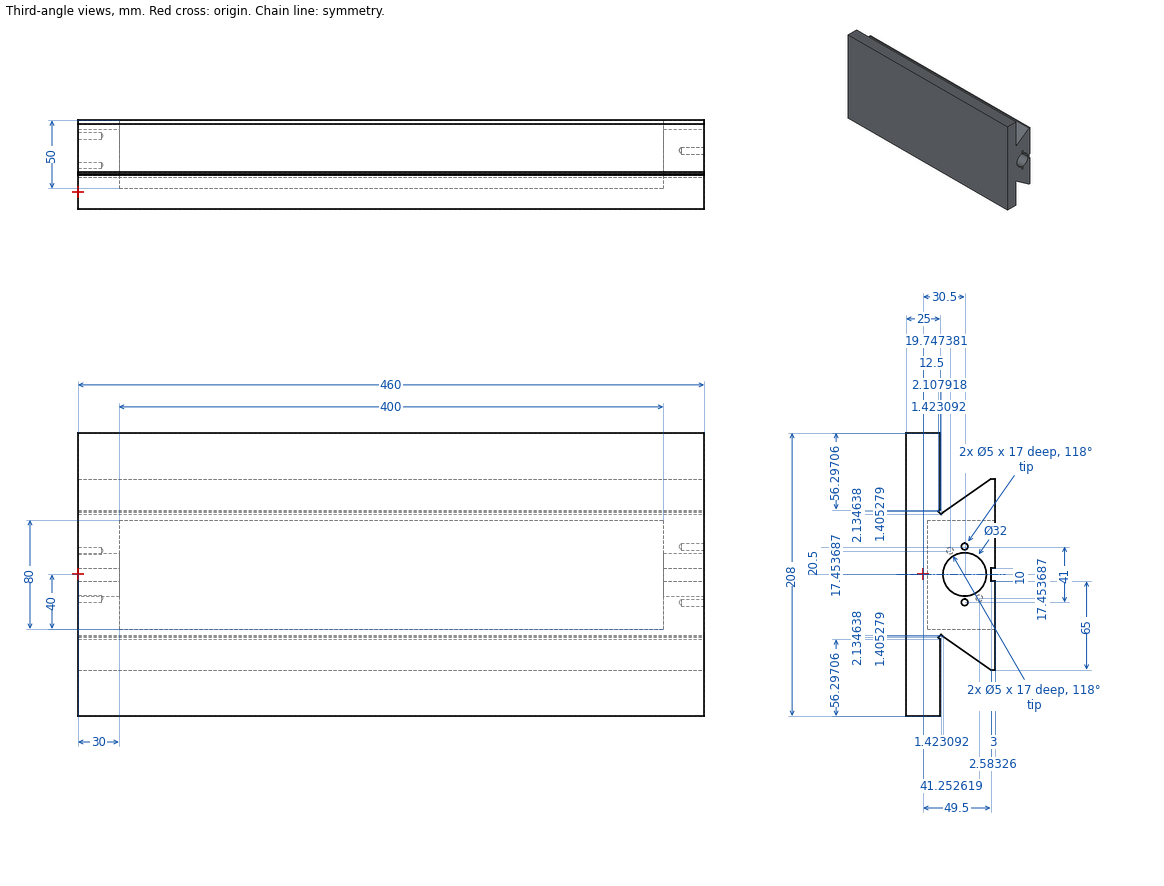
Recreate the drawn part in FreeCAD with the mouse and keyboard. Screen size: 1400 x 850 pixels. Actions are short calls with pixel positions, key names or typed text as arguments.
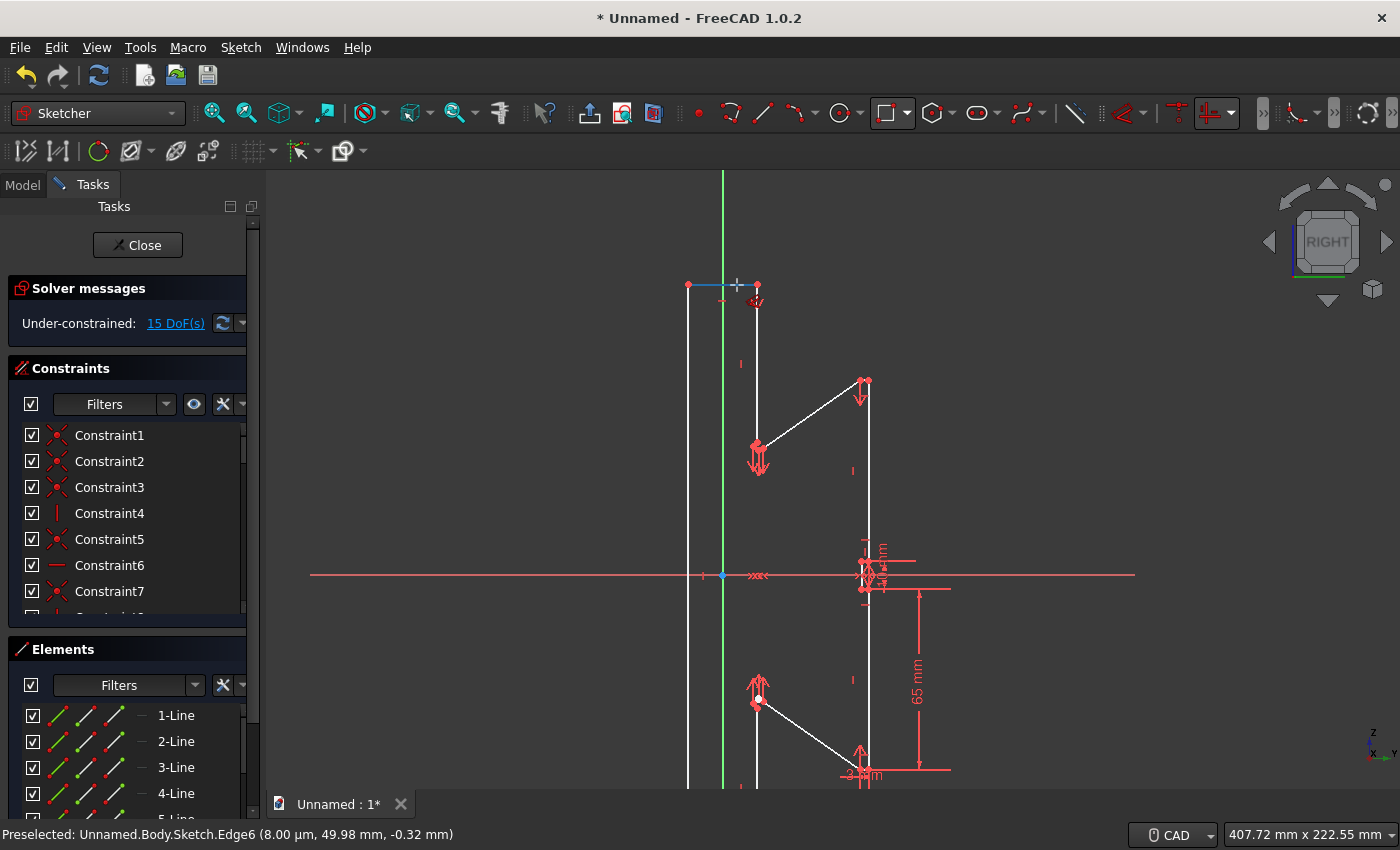
click(736, 285)
click(707, 251)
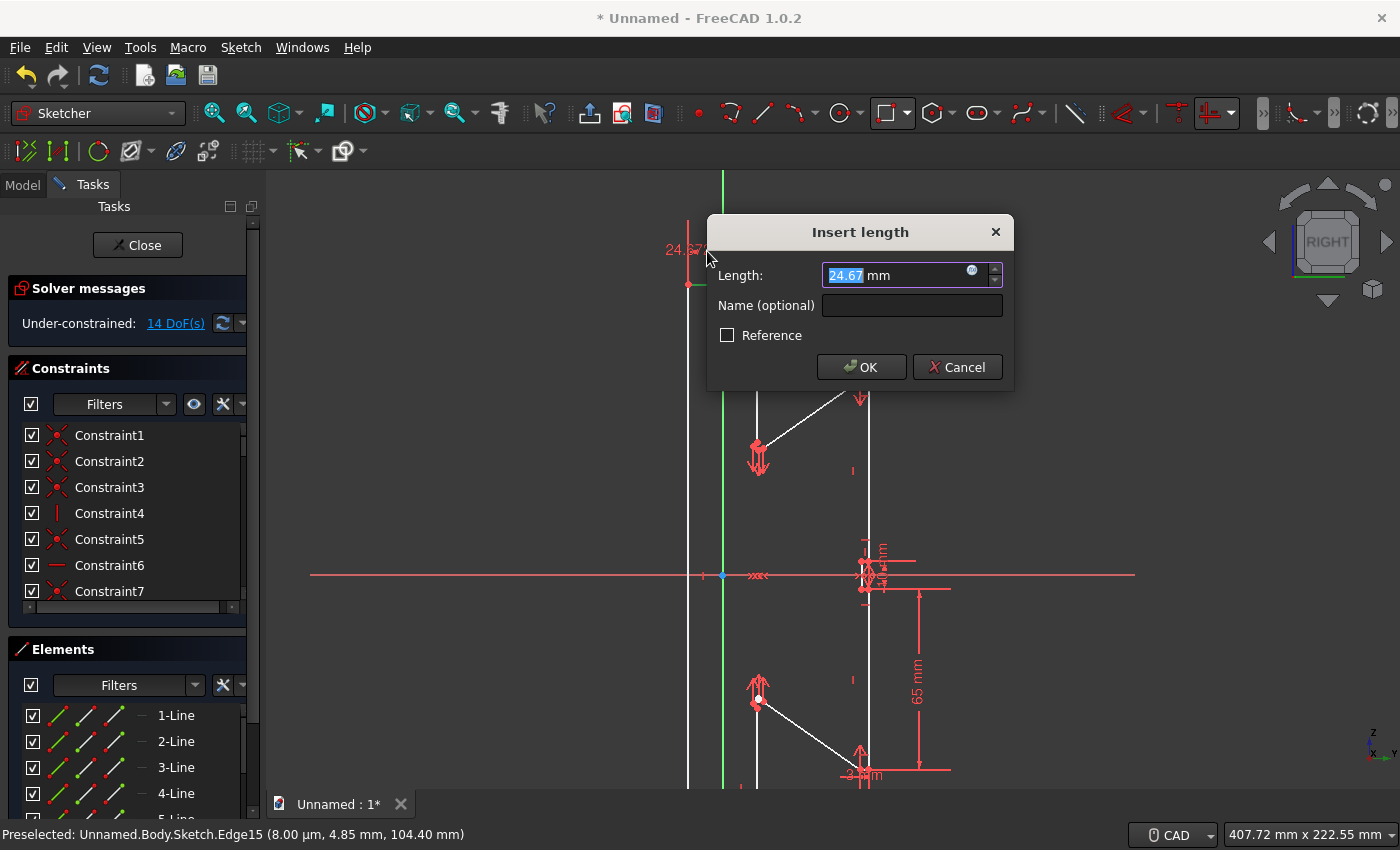
text(25)
key(Return)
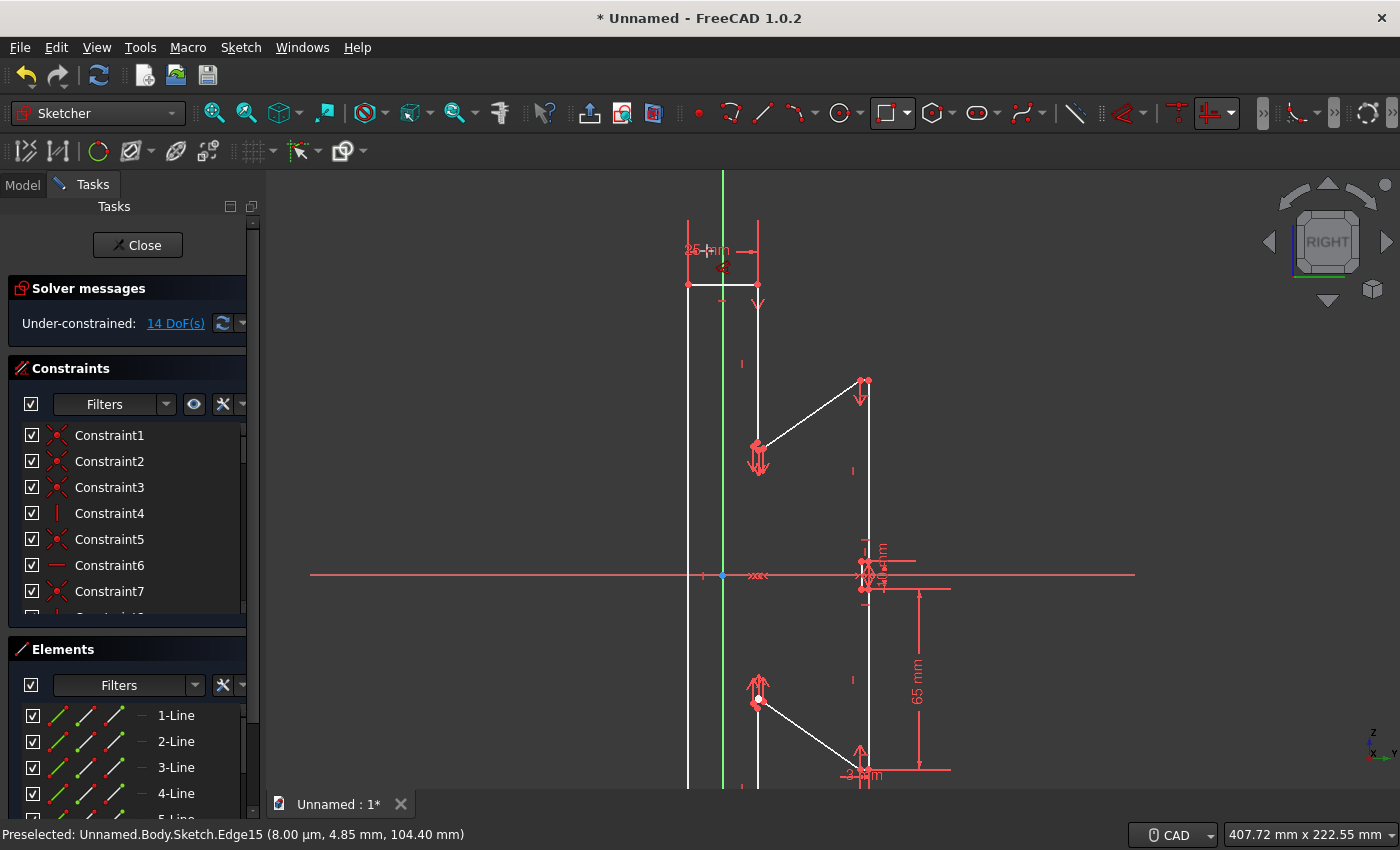
click(688, 459)
click(654, 523)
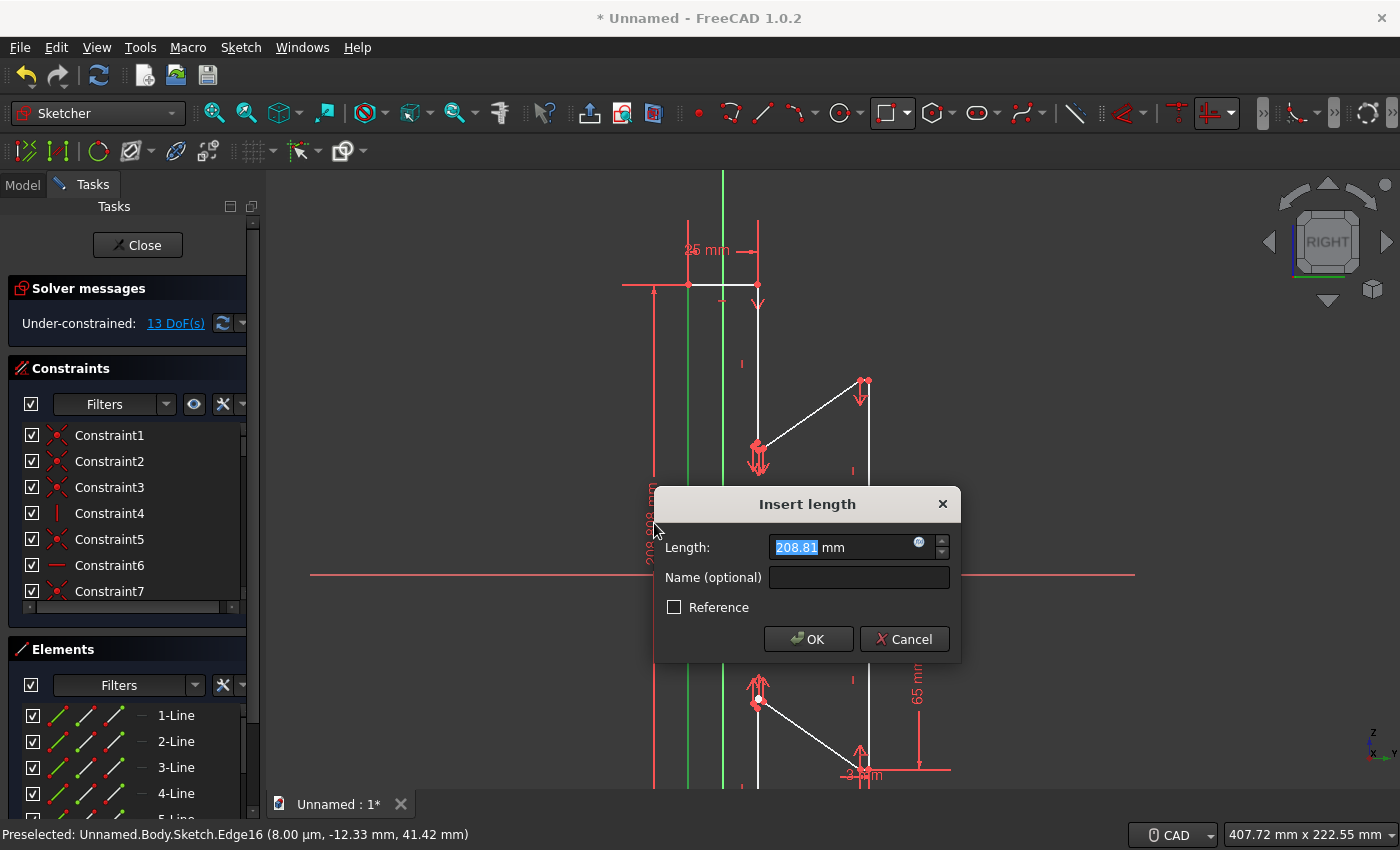
text(208)
key(Return)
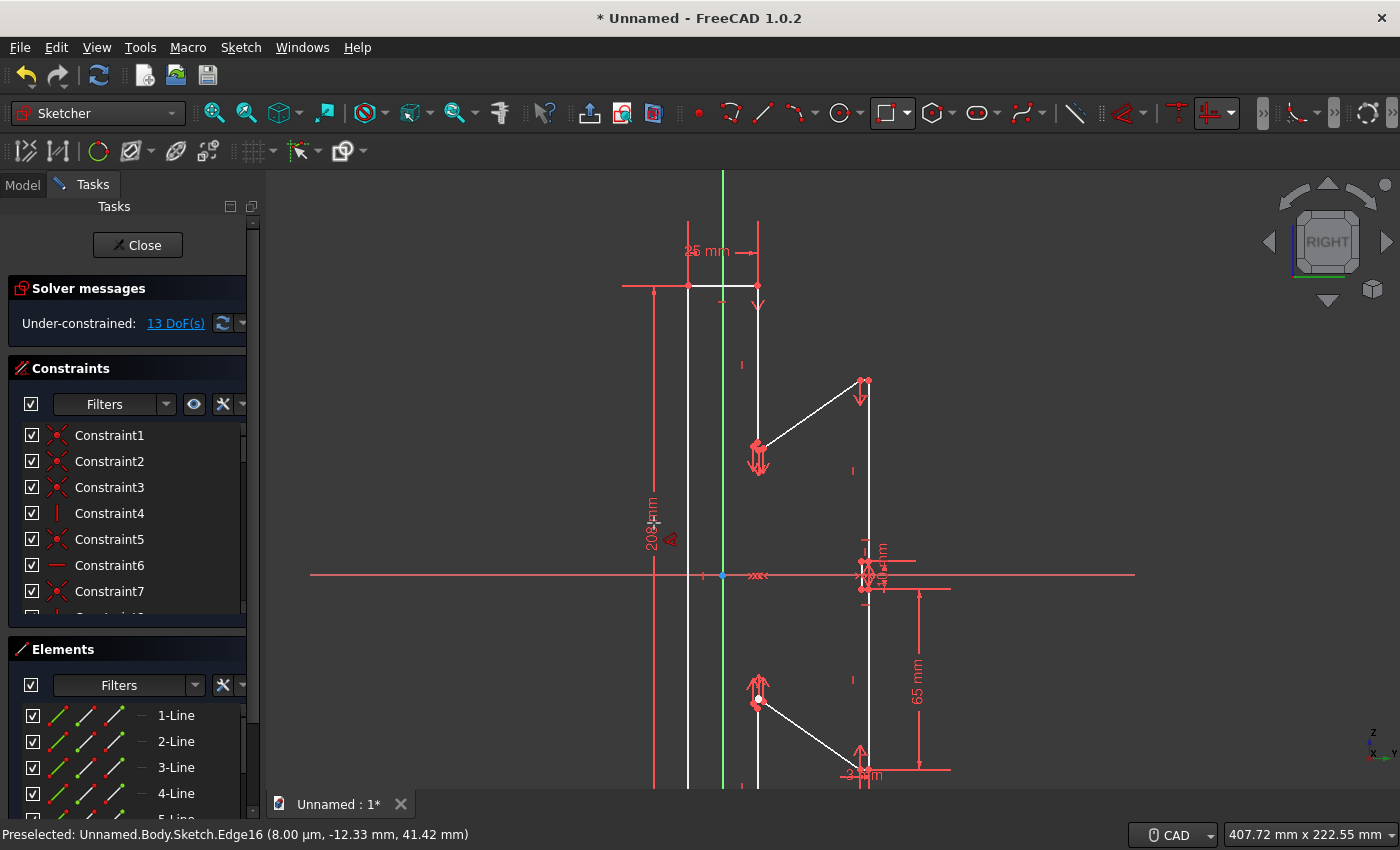
scroll(737, 285, down, 2)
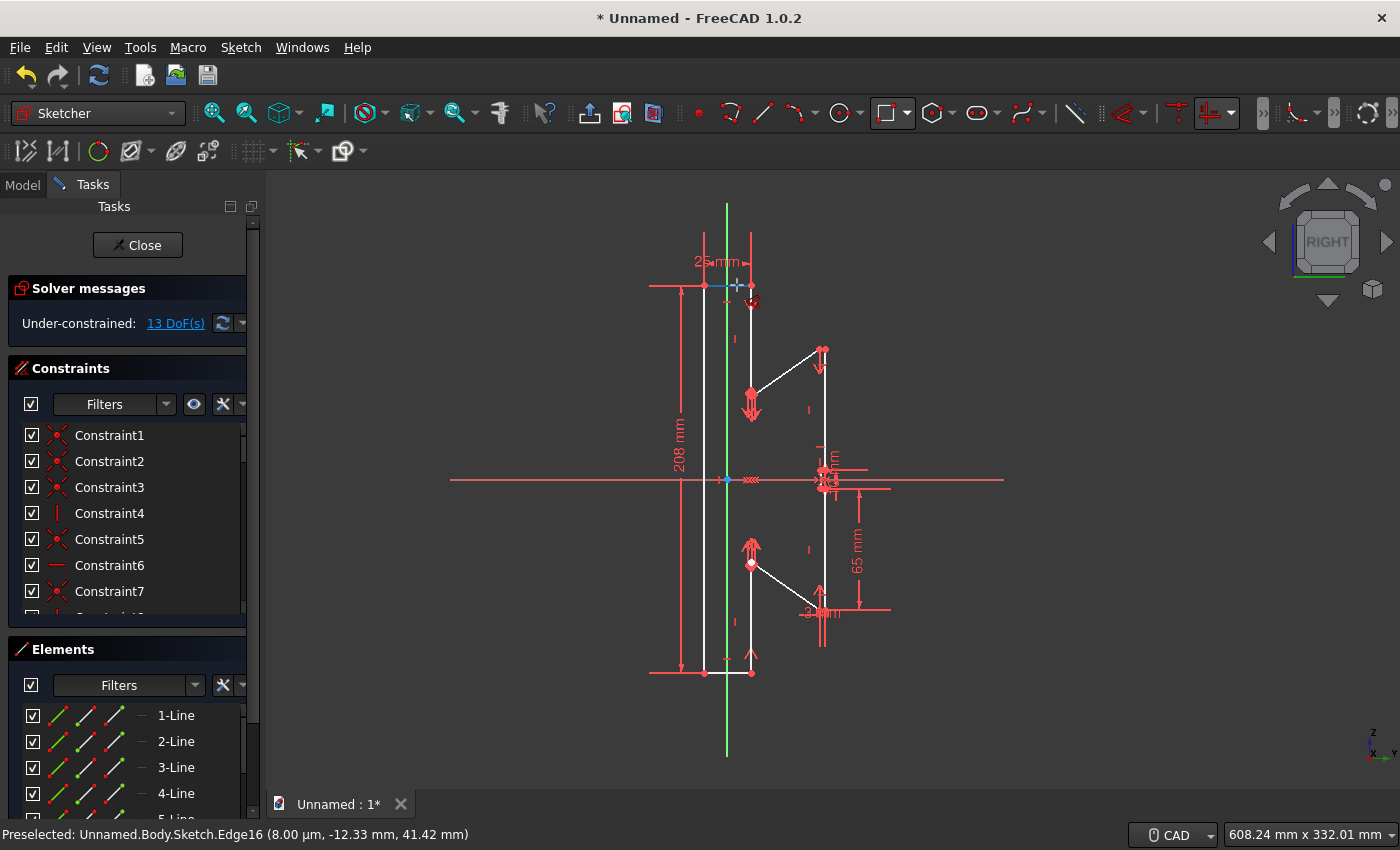
scroll(820, 610, up, 4)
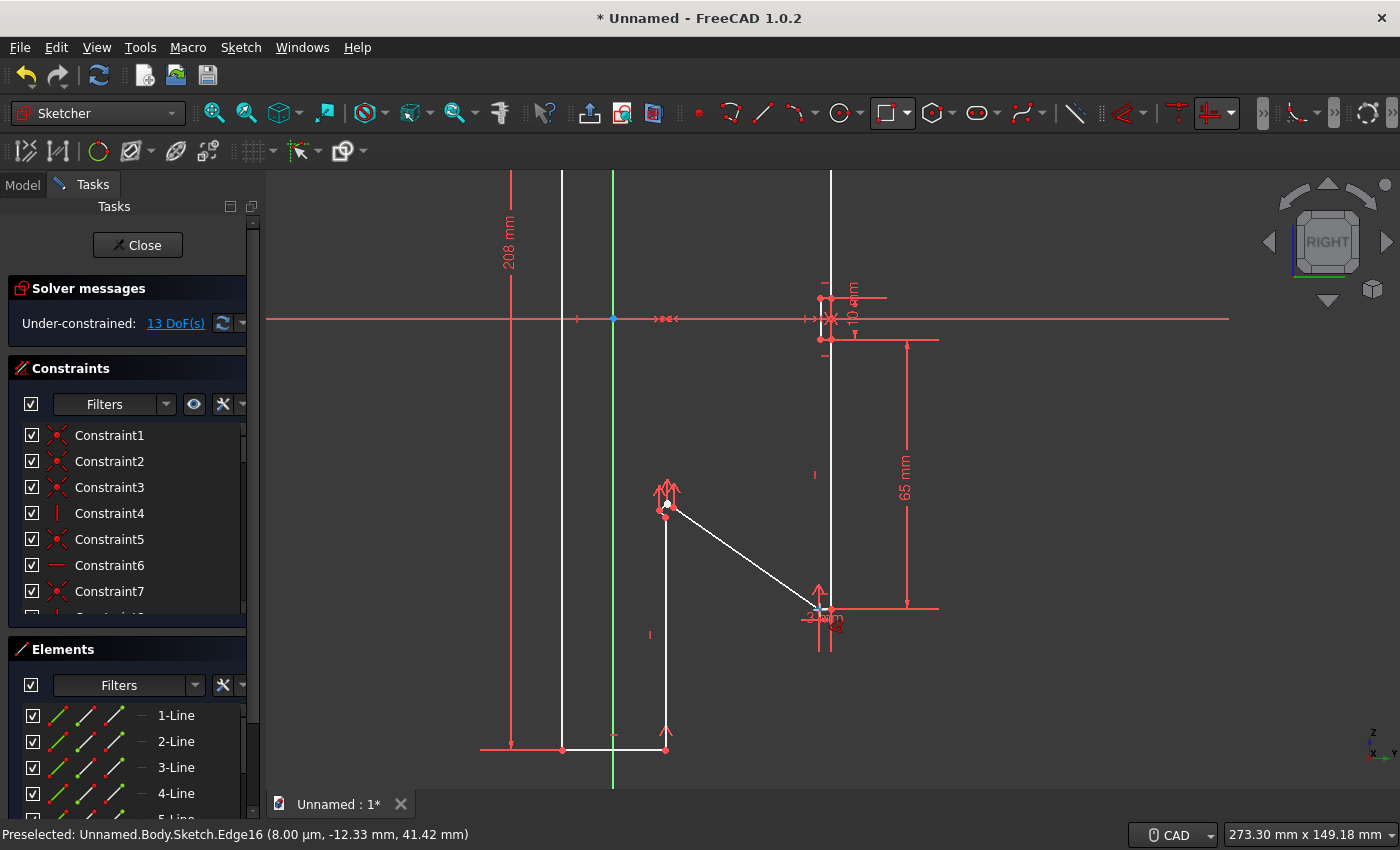
click(819, 609)
click(716, 643)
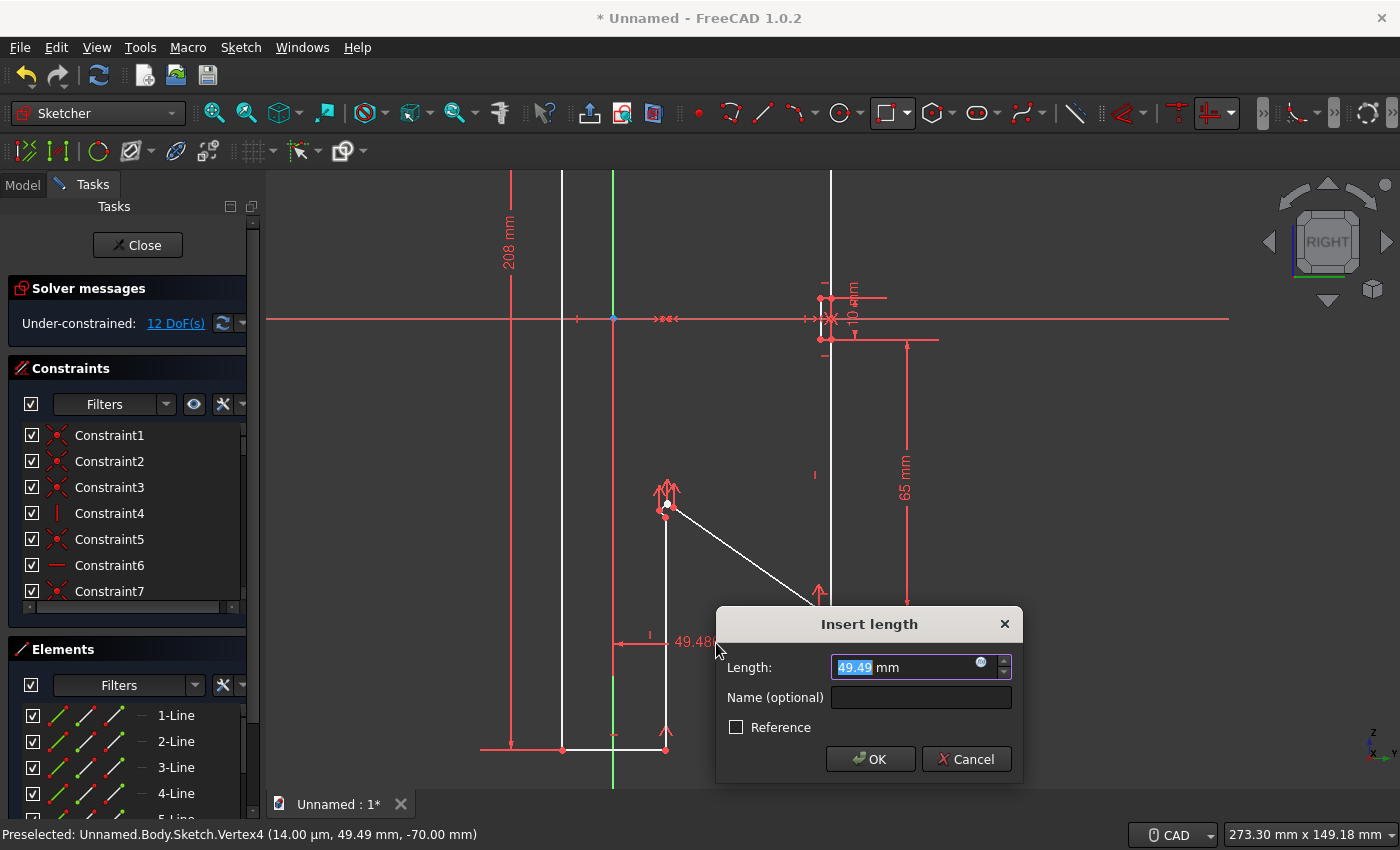
text(49.5)
key(Return)